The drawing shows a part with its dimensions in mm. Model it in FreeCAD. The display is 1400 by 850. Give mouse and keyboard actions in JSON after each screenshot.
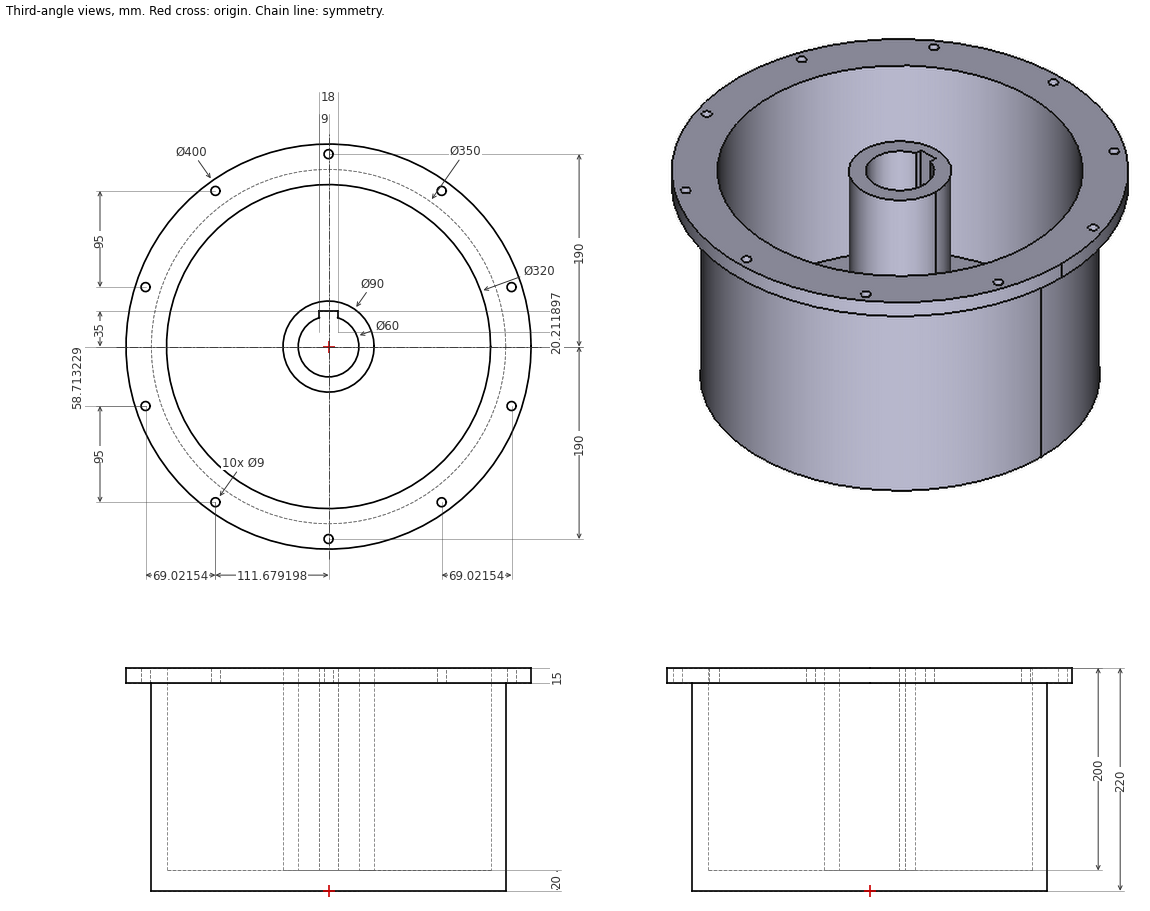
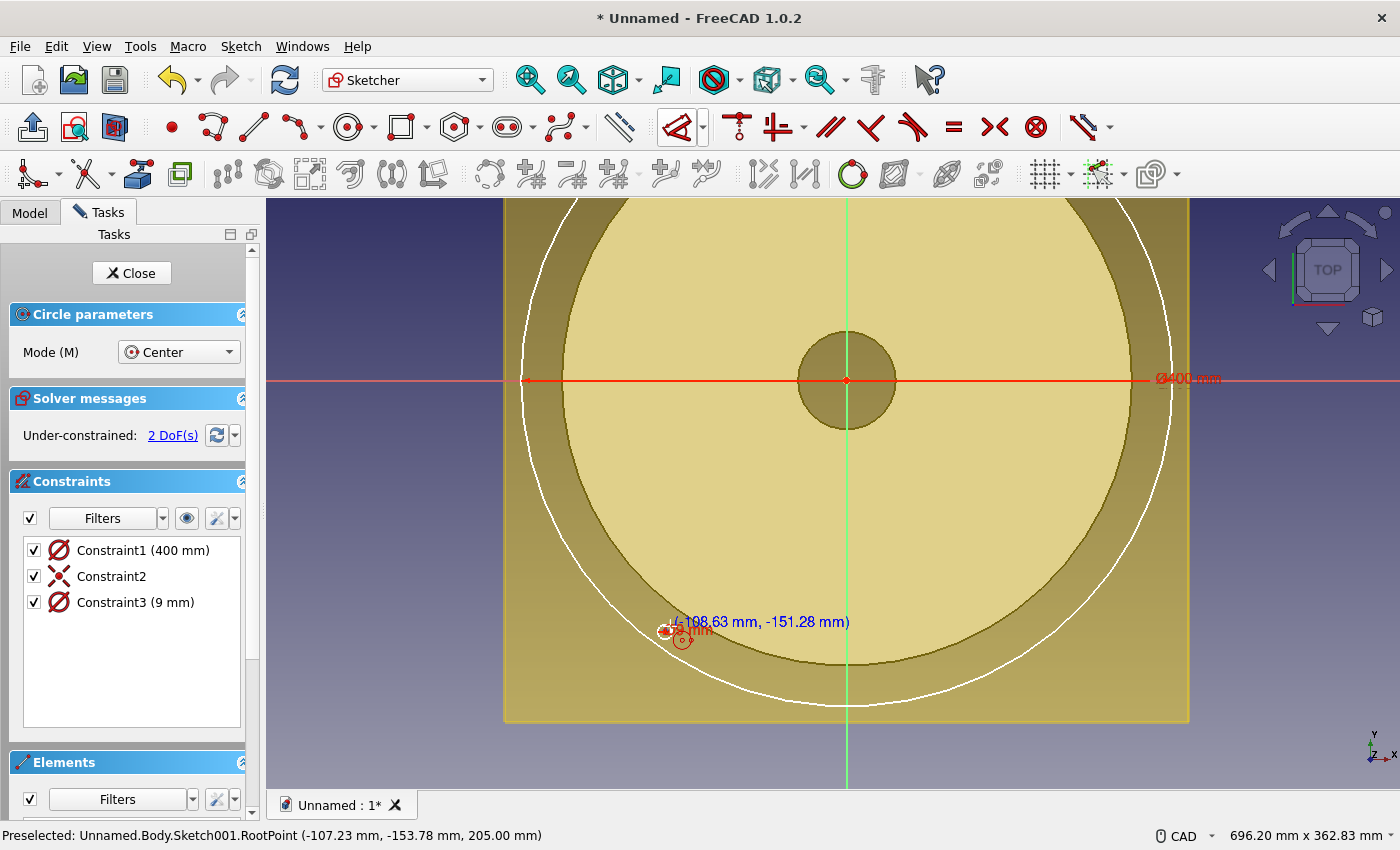
{"action": "scroll", "coordinate": [553, 476], "scroll_direction": "up", "scroll_amount": 6}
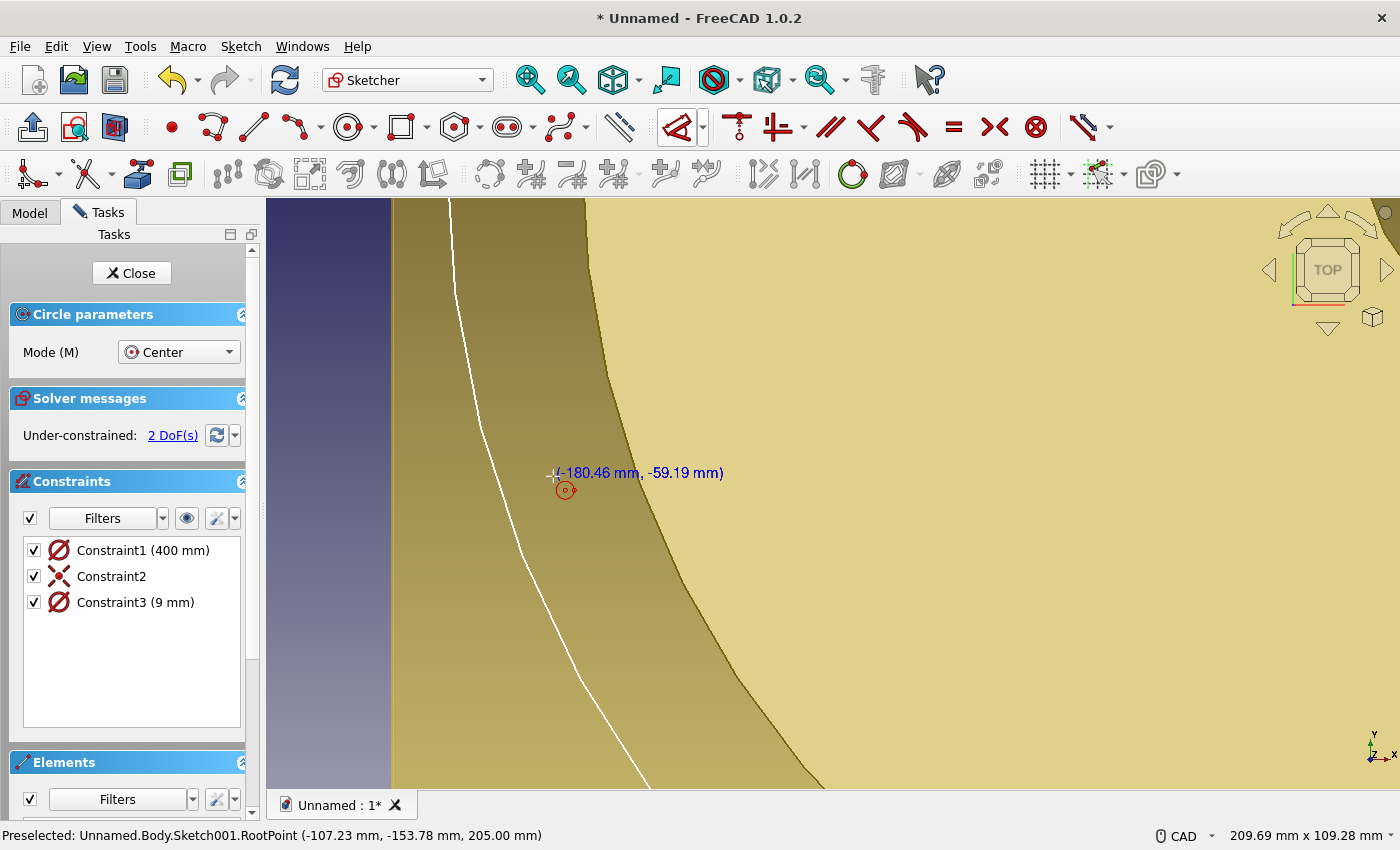
{"action": "scroll", "coordinate": [613, 560], "scroll_direction": "down", "scroll_amount": 9}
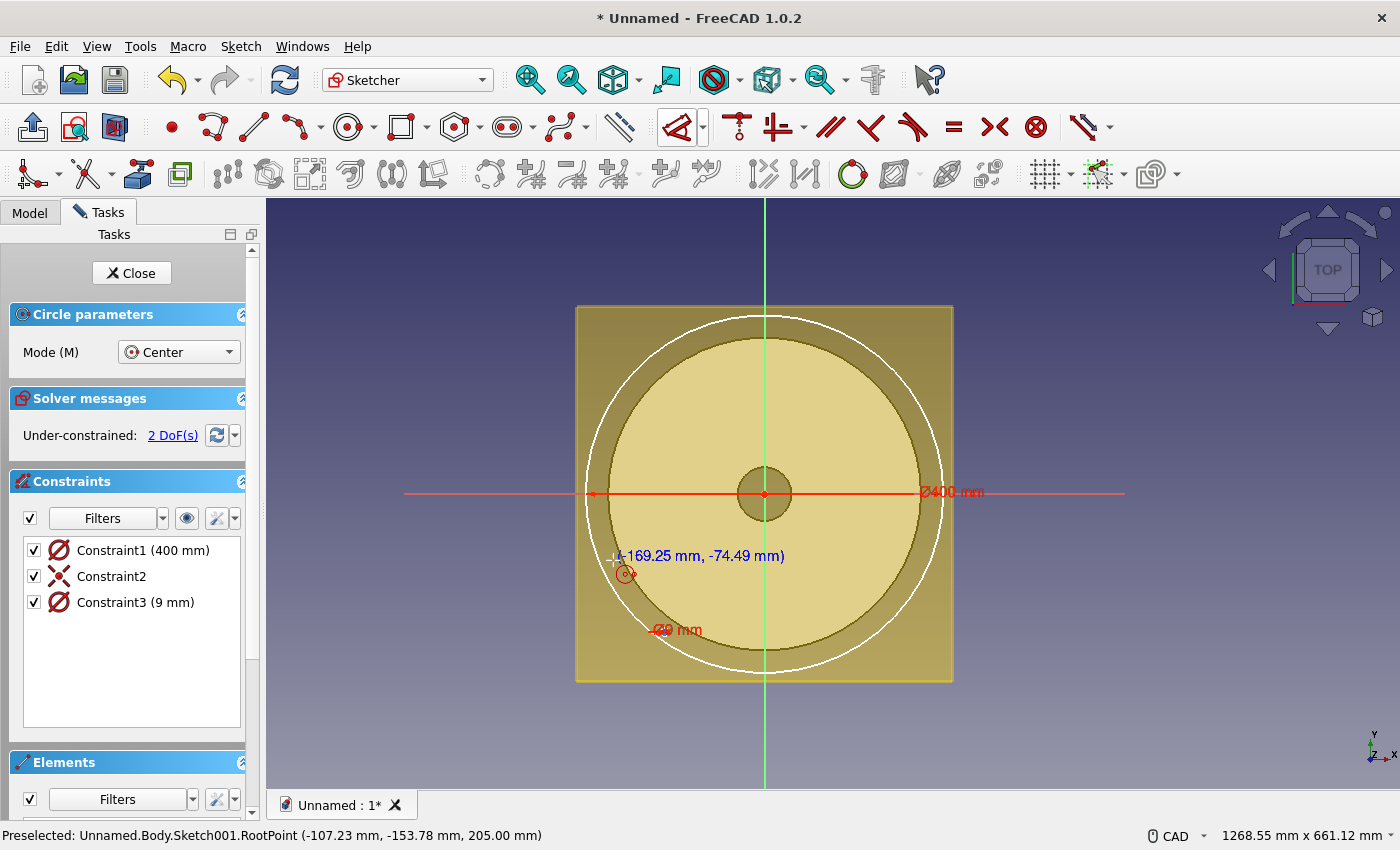
{"action": "scroll", "coordinate": [603, 547], "scroll_direction": "up", "scroll_amount": 3}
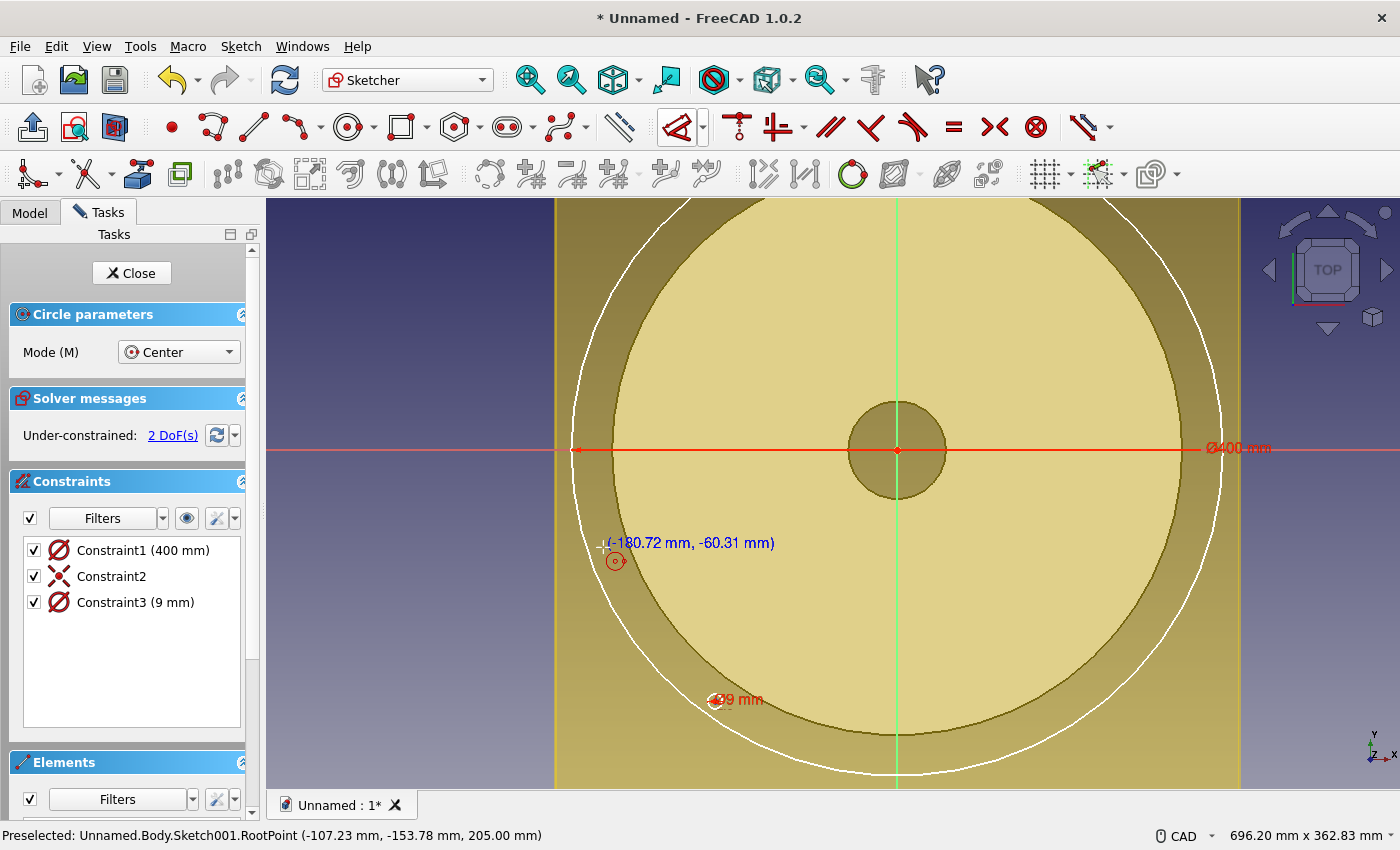
{"action": "left_click", "coordinate": [603, 546]}
{"action": "mouse_move", "coordinate": [608, 541]}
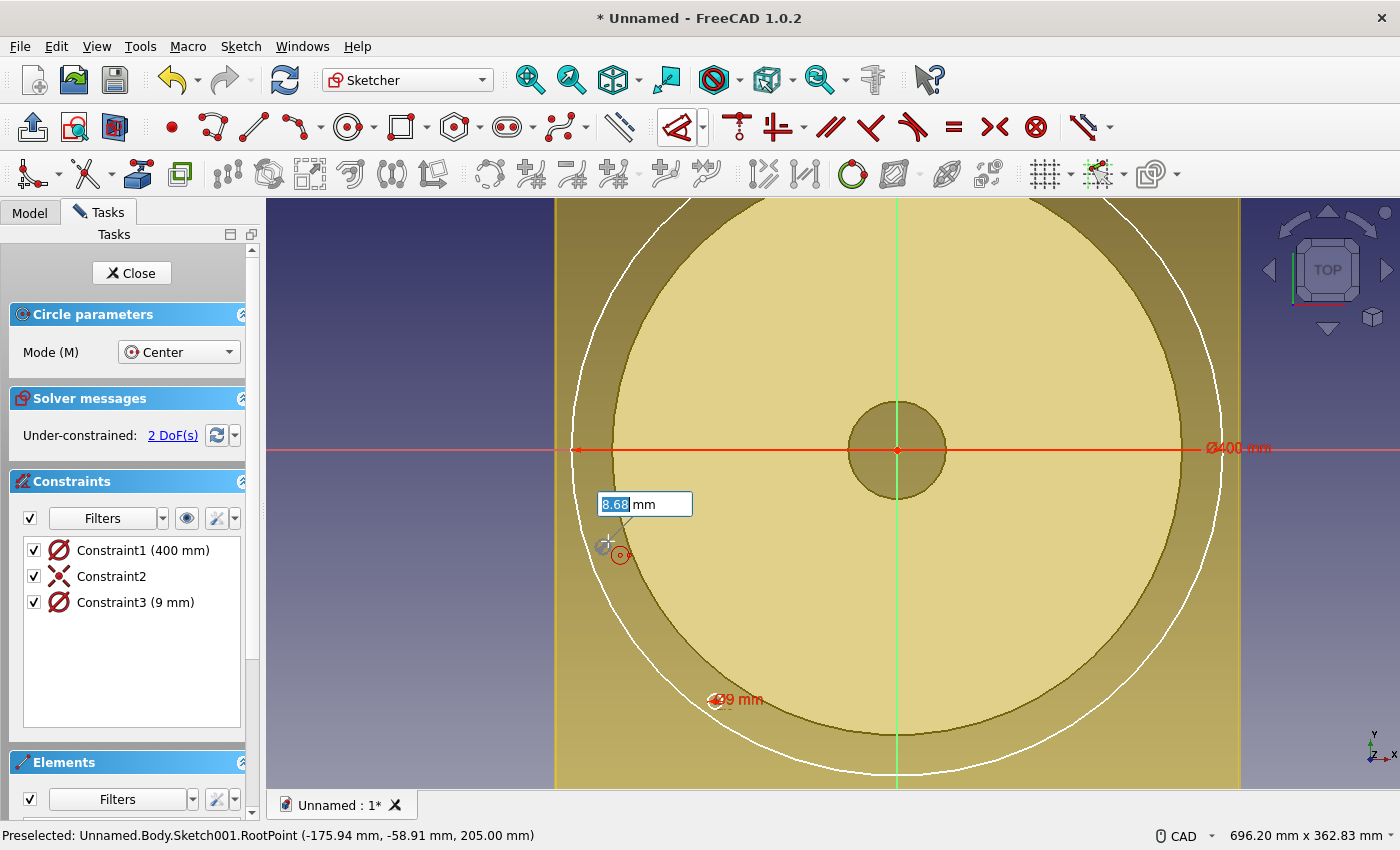
{"action": "type", "text": "9"}
{"action": "key", "text": "Return"}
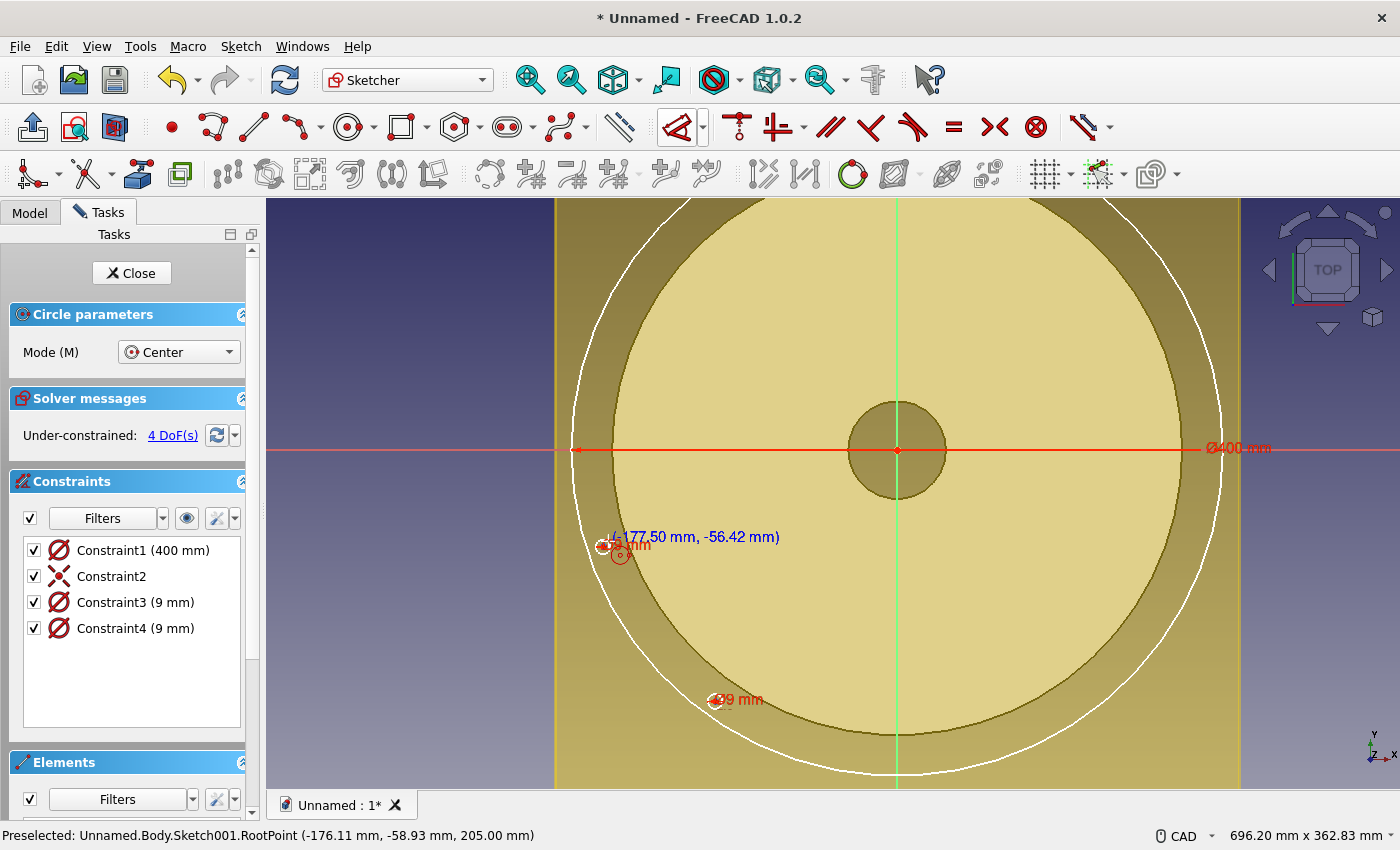
{"action": "scroll", "coordinate": [897, 760], "scroll_direction": "up", "scroll_amount": 6}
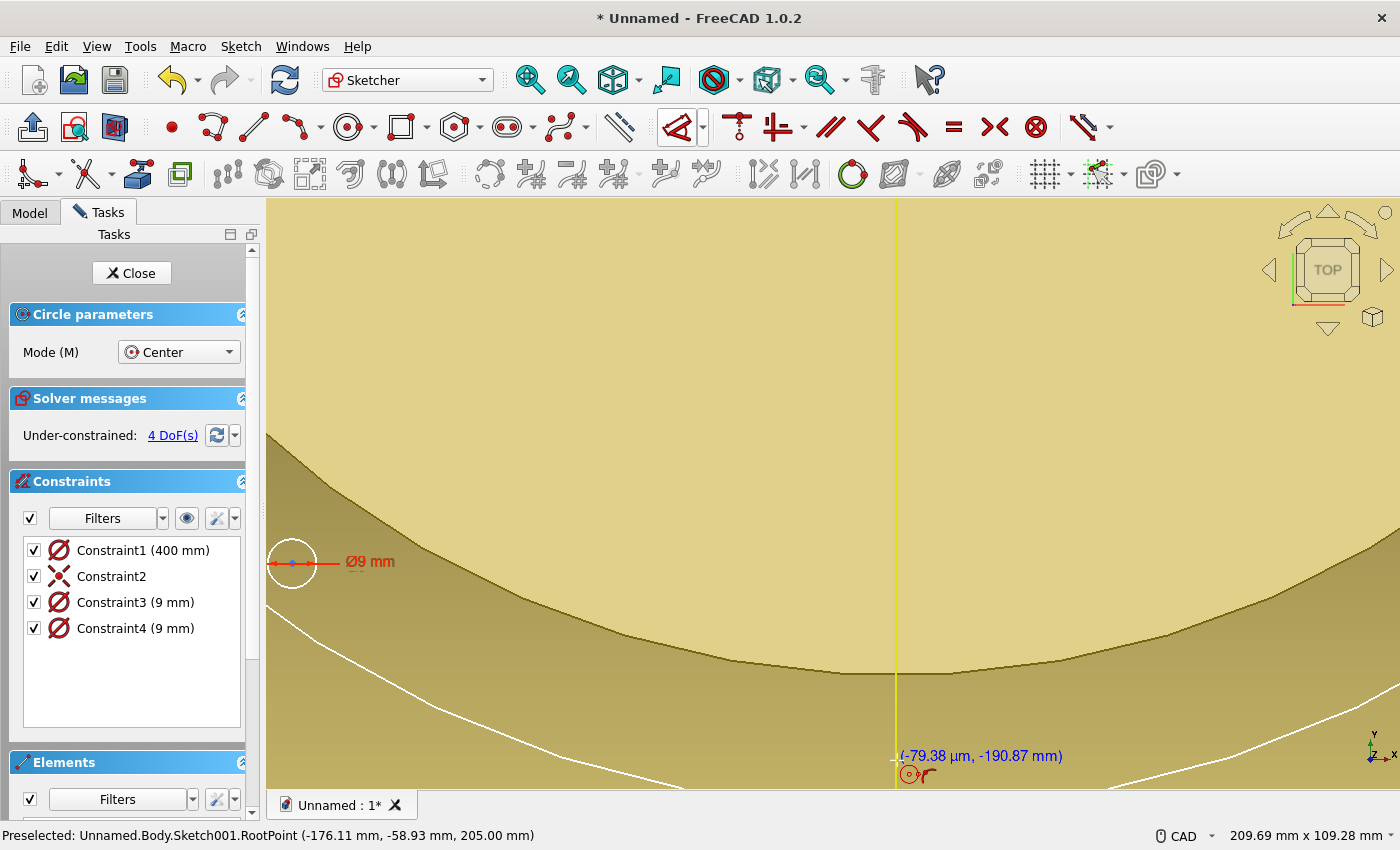
{"action": "scroll", "coordinate": [738, 645], "scroll_direction": "down", "scroll_amount": 9}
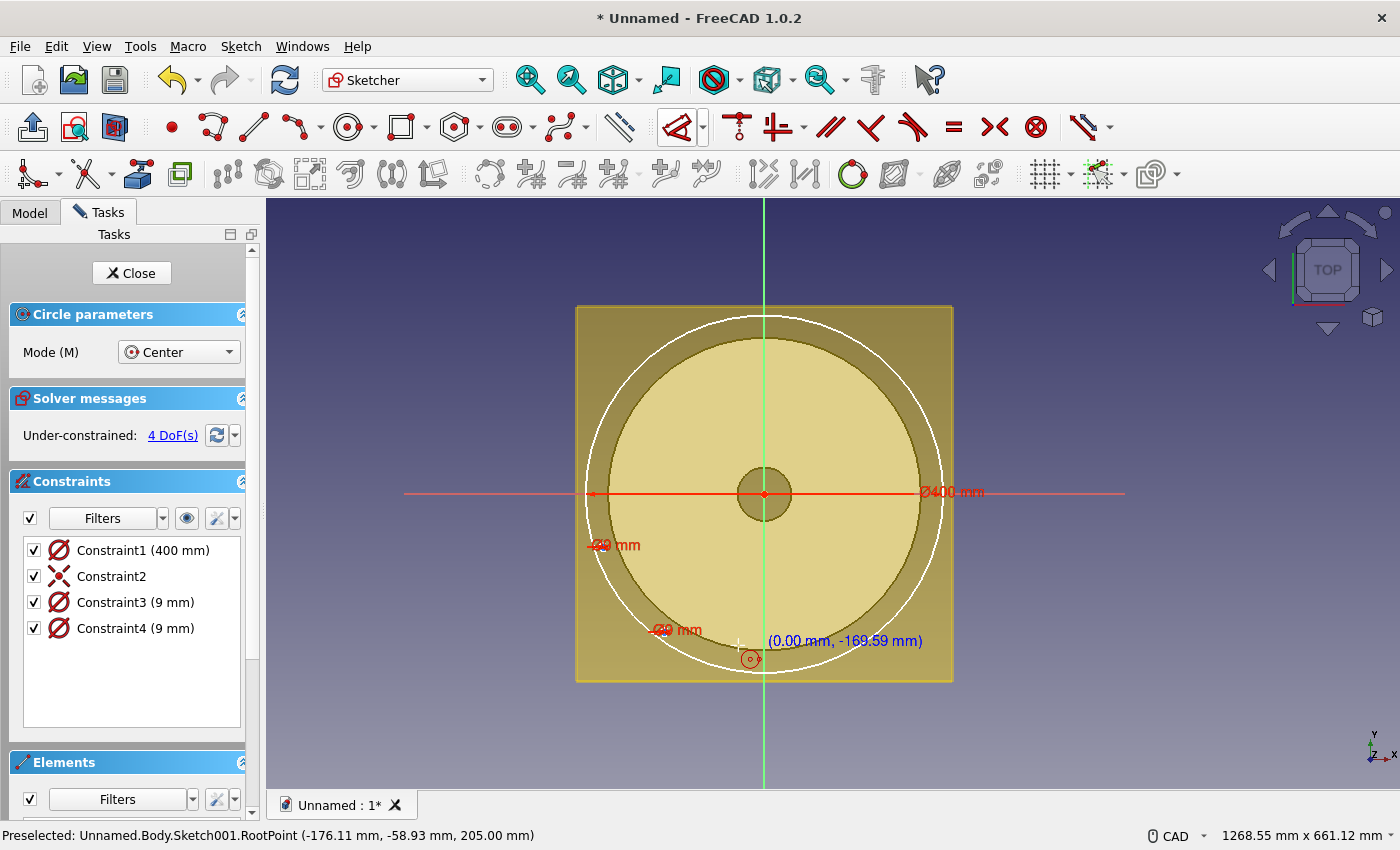
{"action": "scroll", "coordinate": [764, 664], "scroll_direction": "up", "scroll_amount": 3}